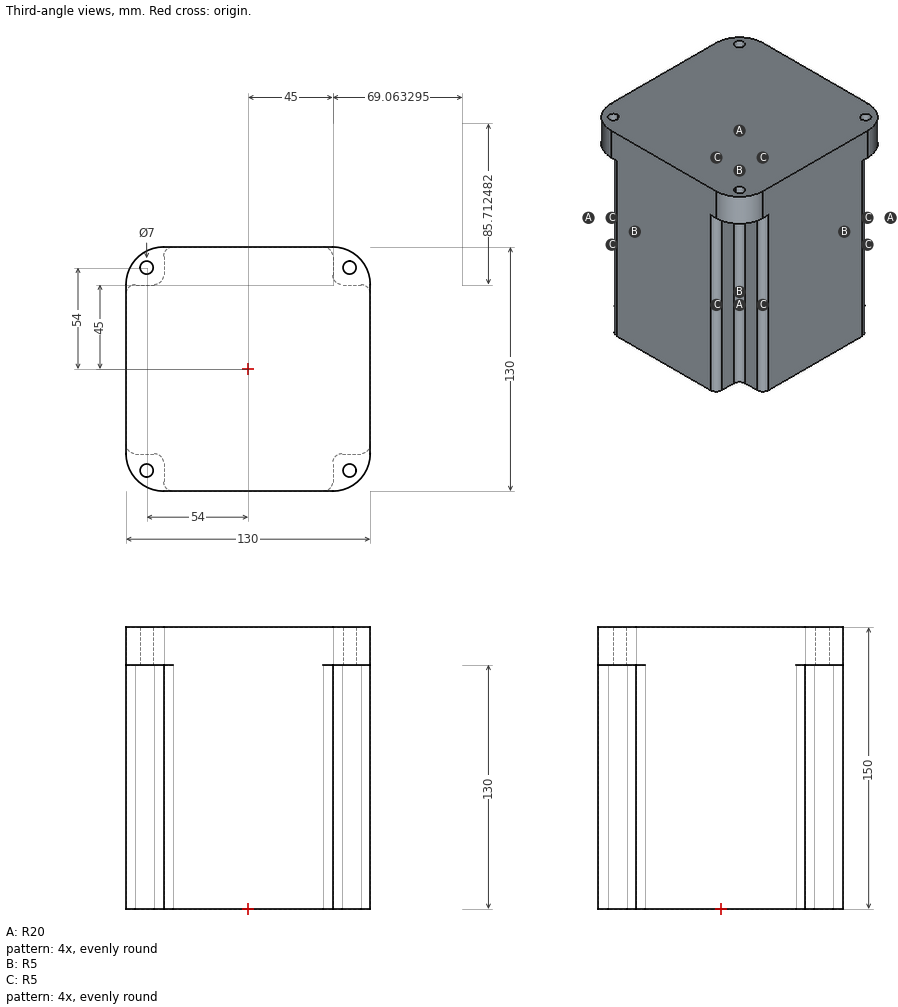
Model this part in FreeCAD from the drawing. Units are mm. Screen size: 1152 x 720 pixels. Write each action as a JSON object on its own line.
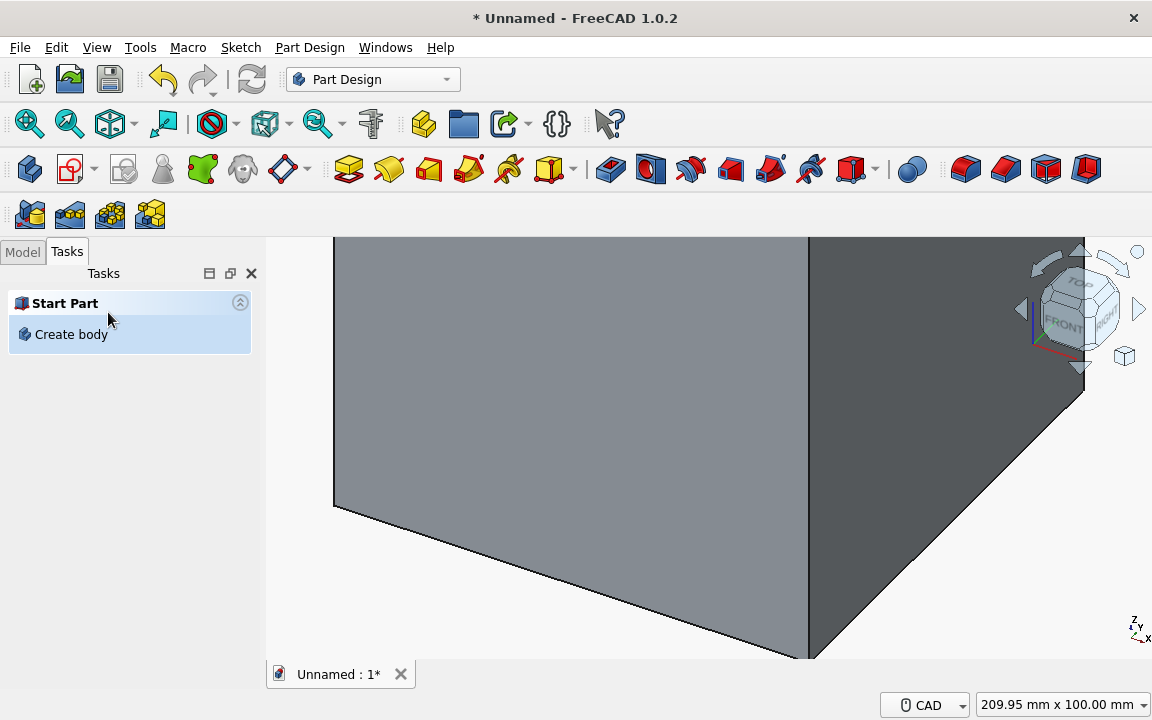
{"action": "key", "text": "v f"}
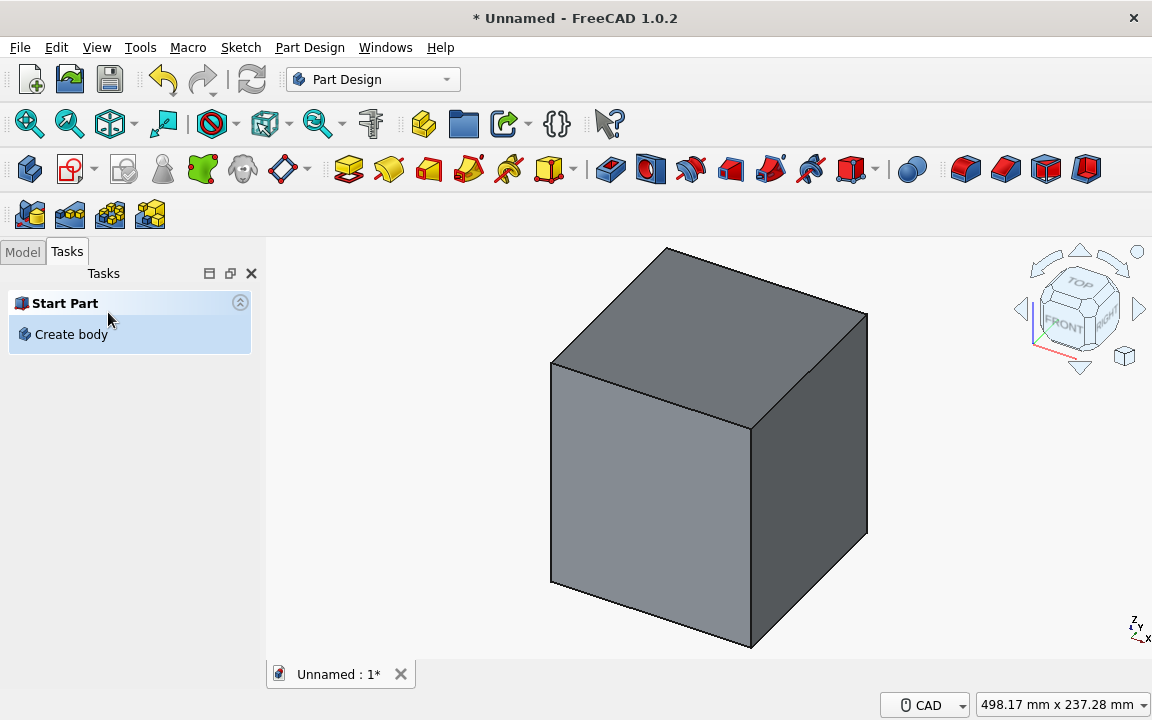
{"action": "left_click", "coordinate": [751, 538]}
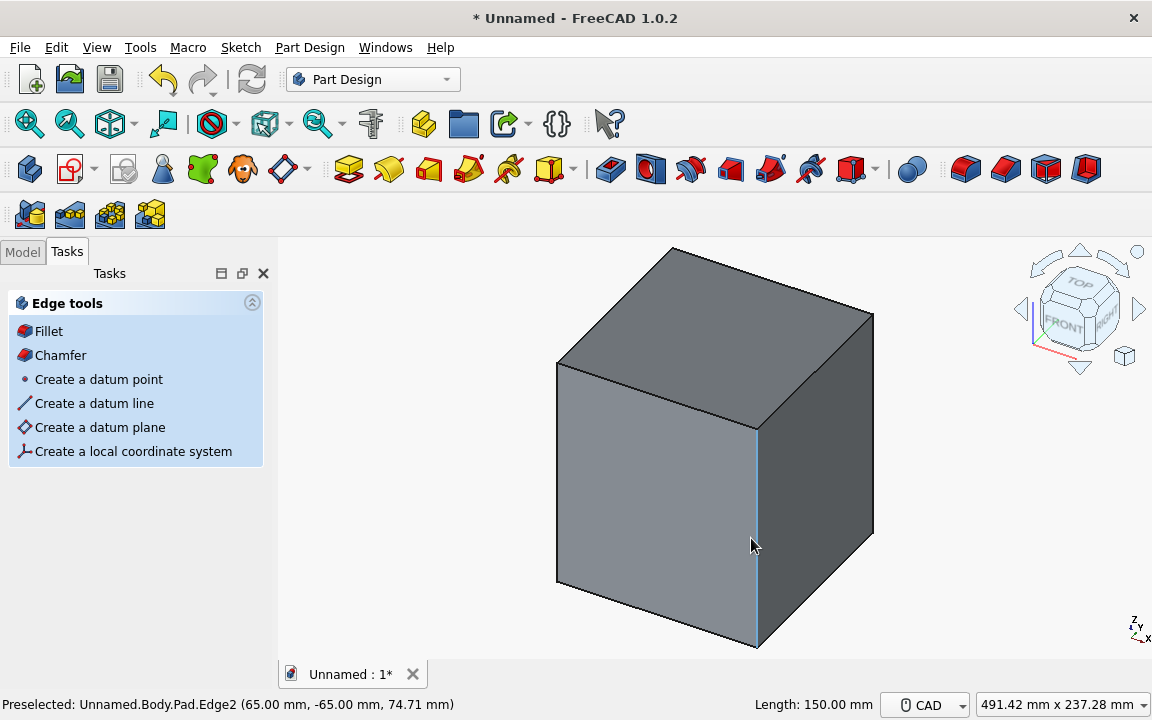
{"action": "key", "text": "0"}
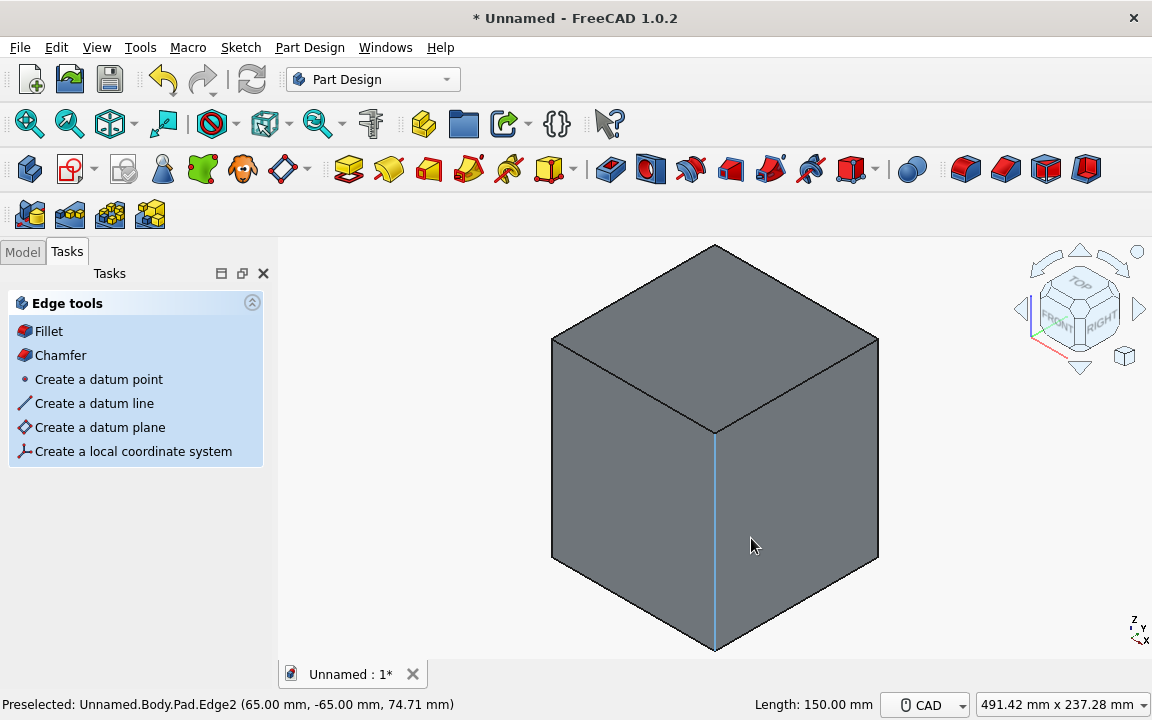
{"action": "key", "text": "2"}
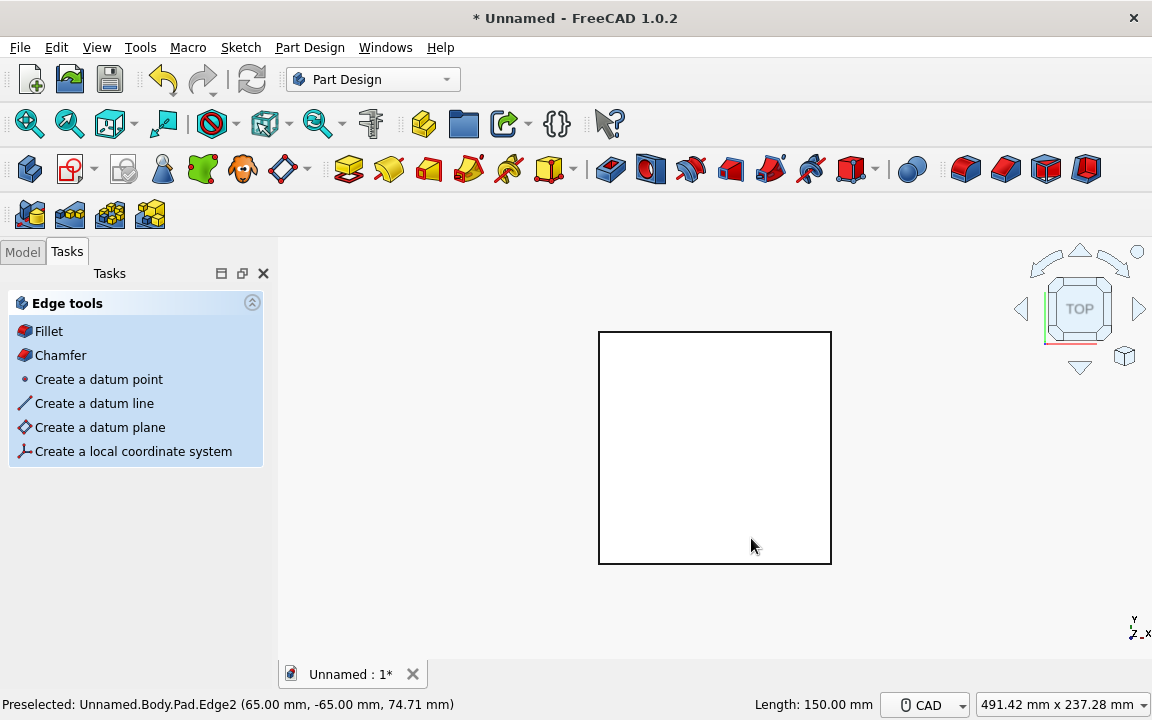
{"action": "key", "text": "1"}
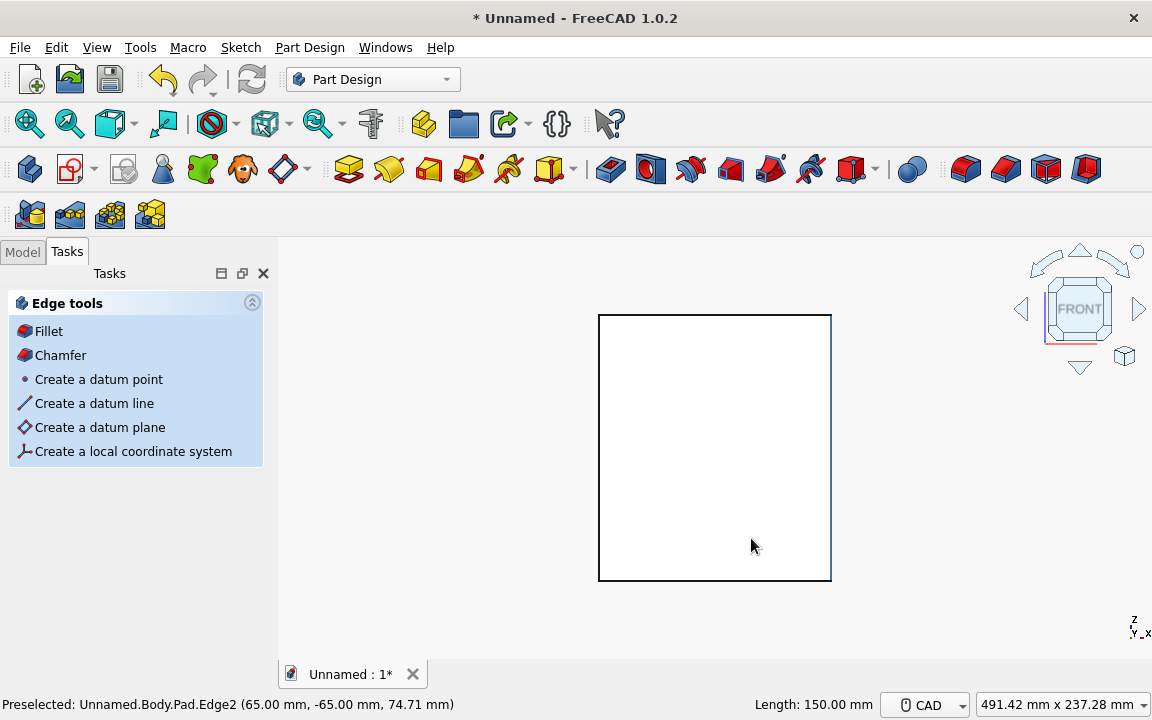
{"action": "left_click", "coordinate": [599, 447], "text": "ctrl"}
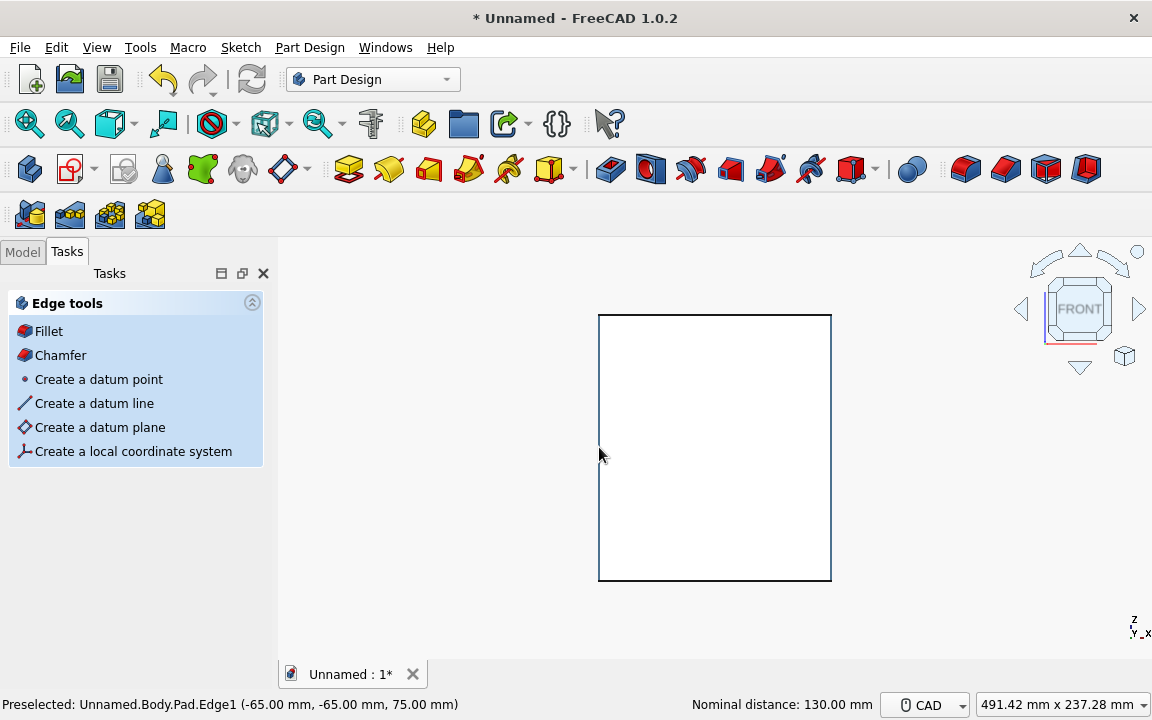
{"action": "key", "text": "3"}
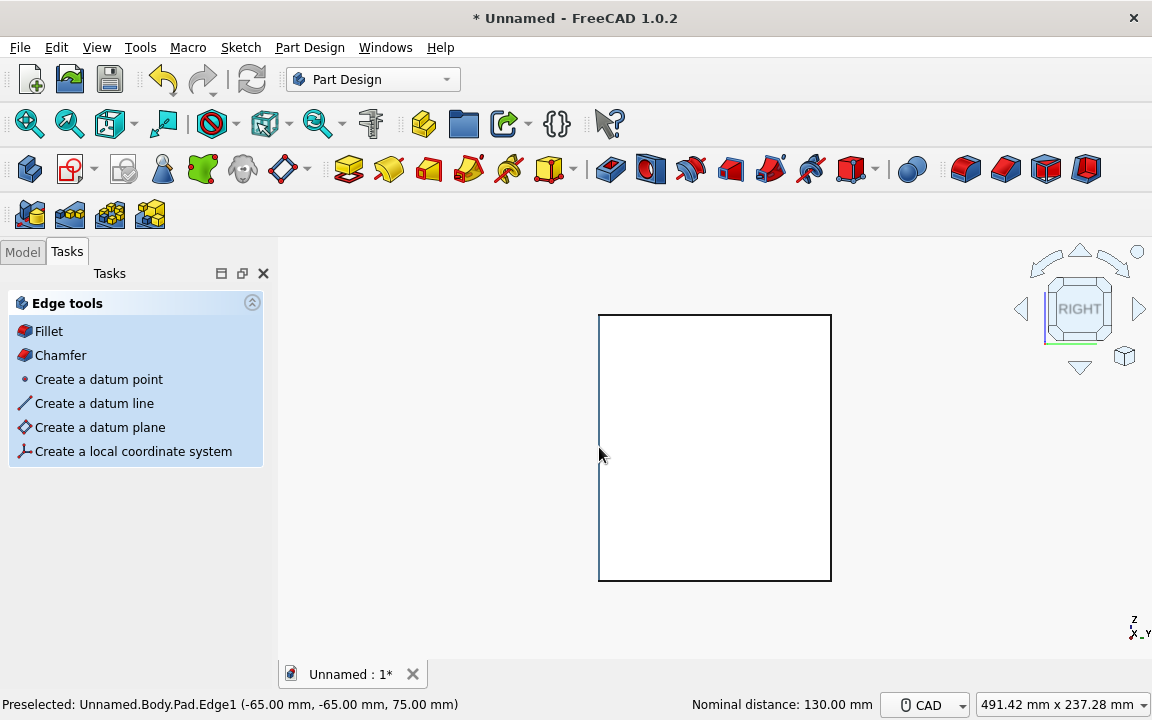
{"action": "left_click", "coordinate": [831, 447], "text": "ctrl"}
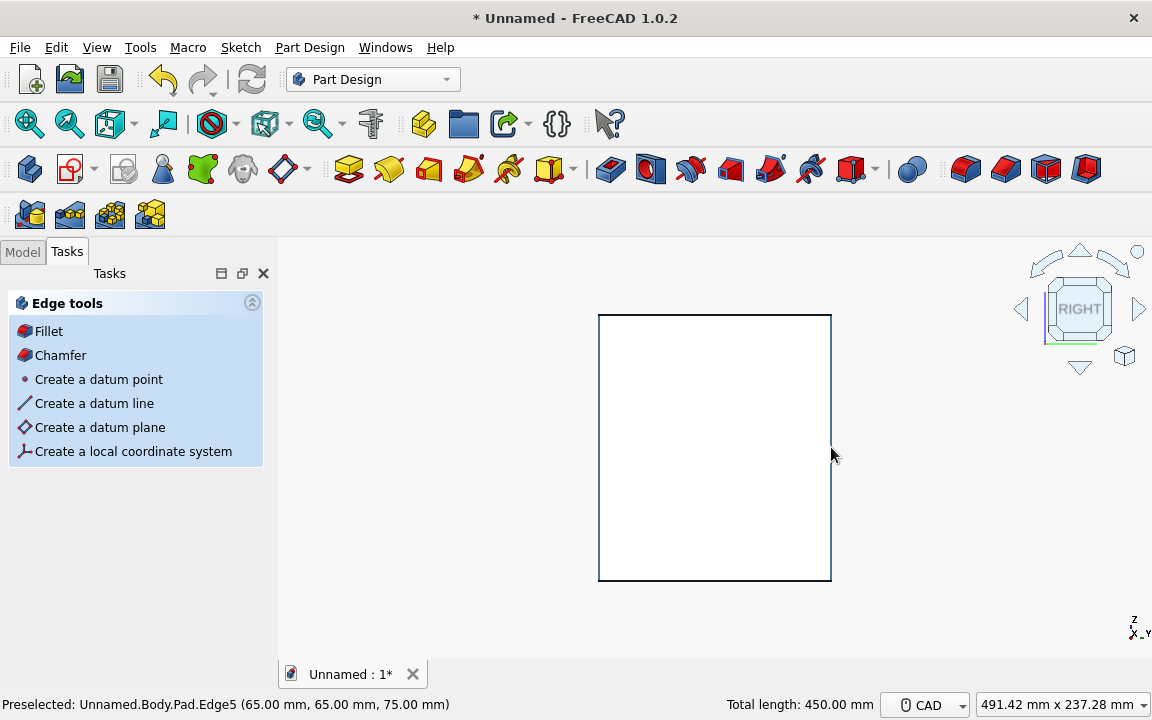
{"action": "key", "text": "5"}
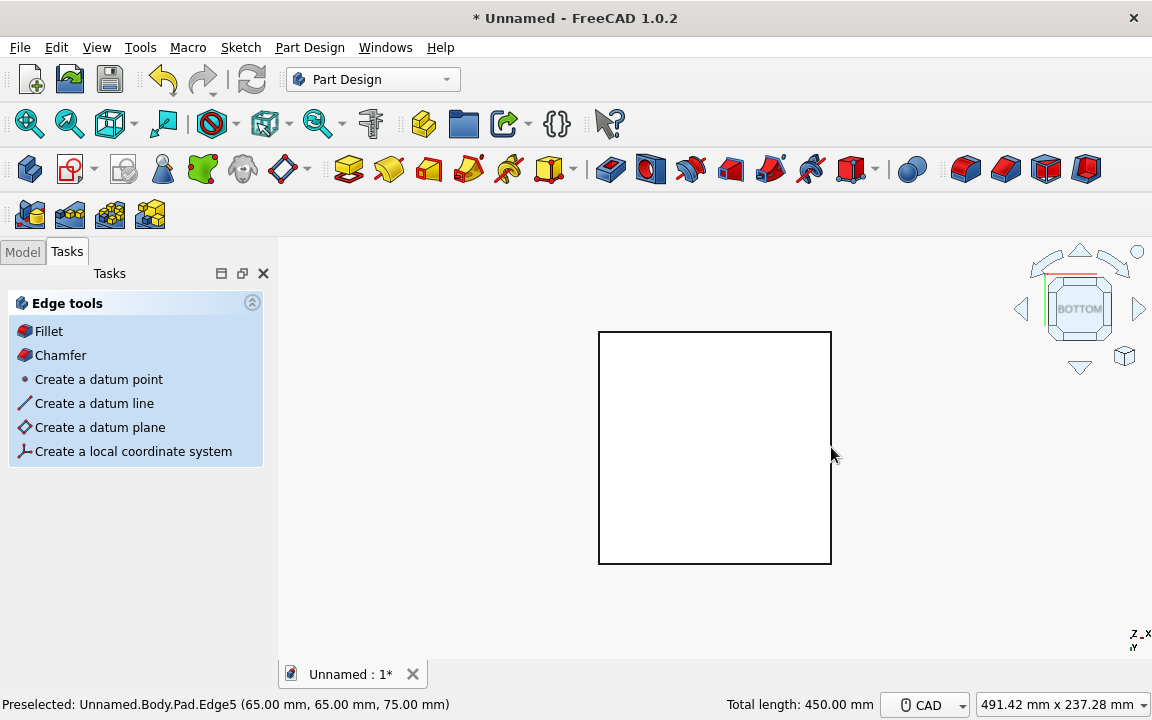
{"action": "key", "text": "4"}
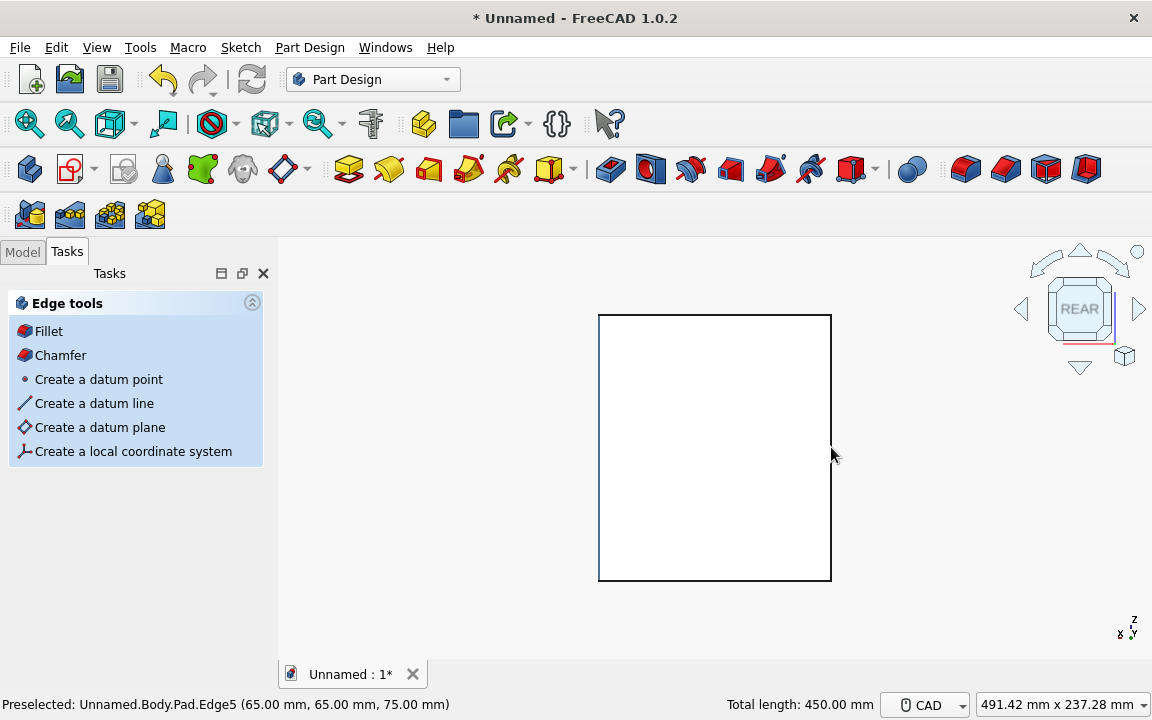
{"action": "left_click", "coordinate": [831, 447], "text": "ctrl"}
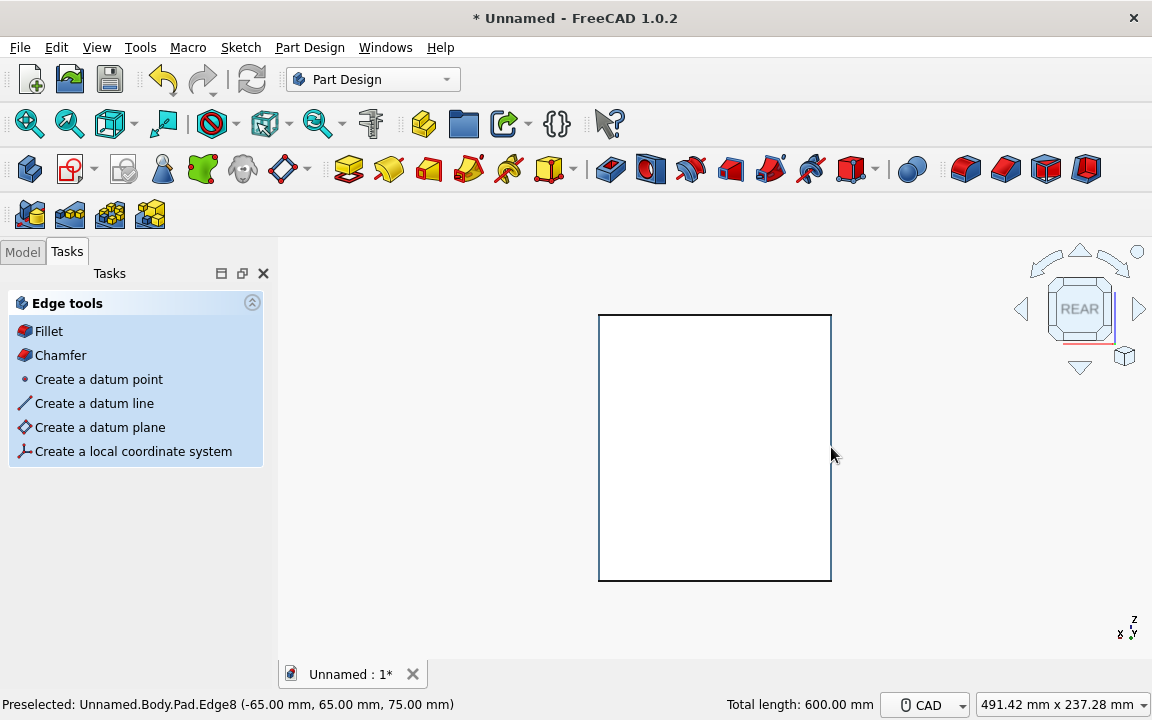
{"action": "left_click", "coordinate": [966, 170]}